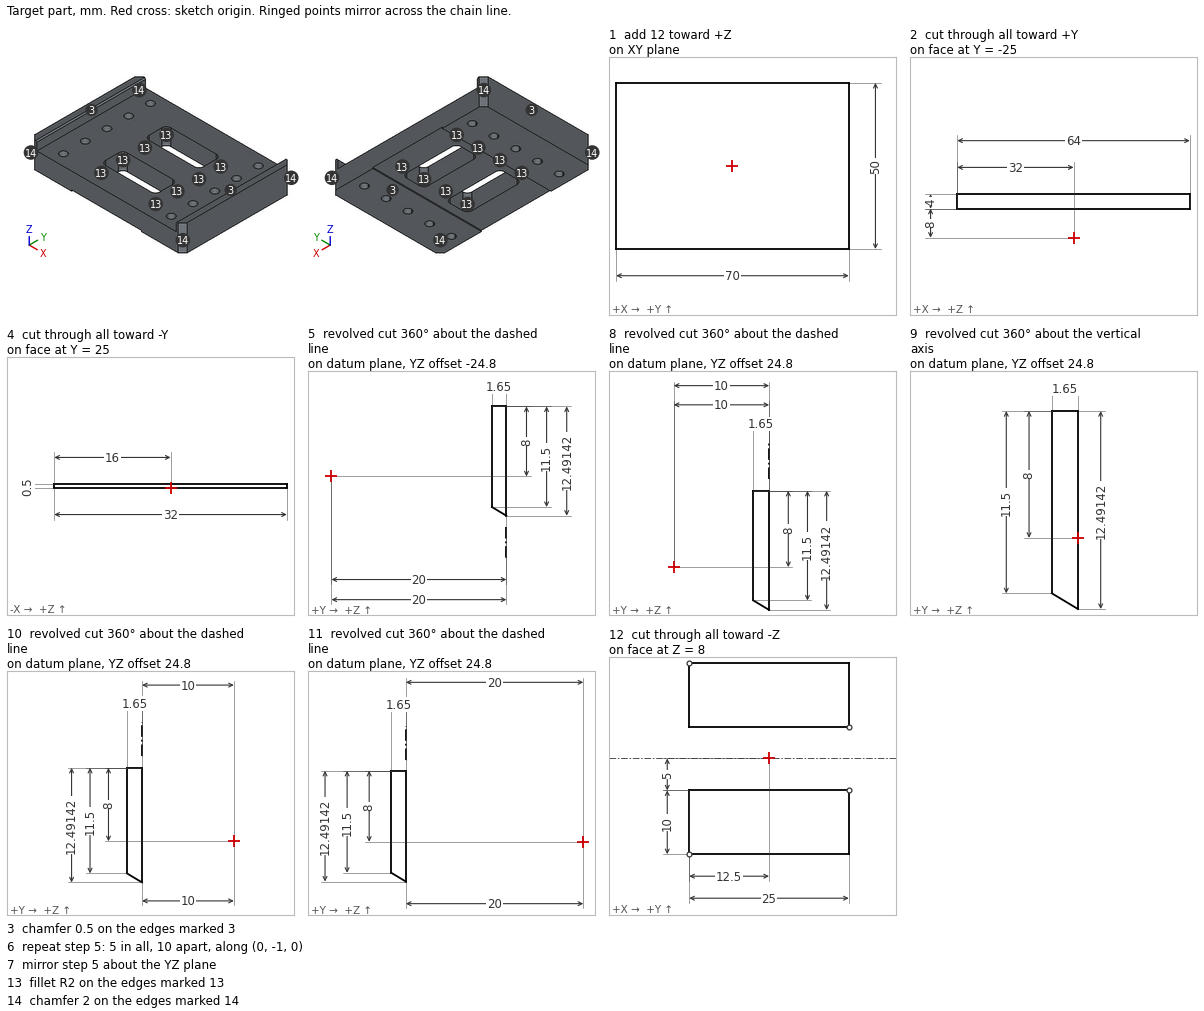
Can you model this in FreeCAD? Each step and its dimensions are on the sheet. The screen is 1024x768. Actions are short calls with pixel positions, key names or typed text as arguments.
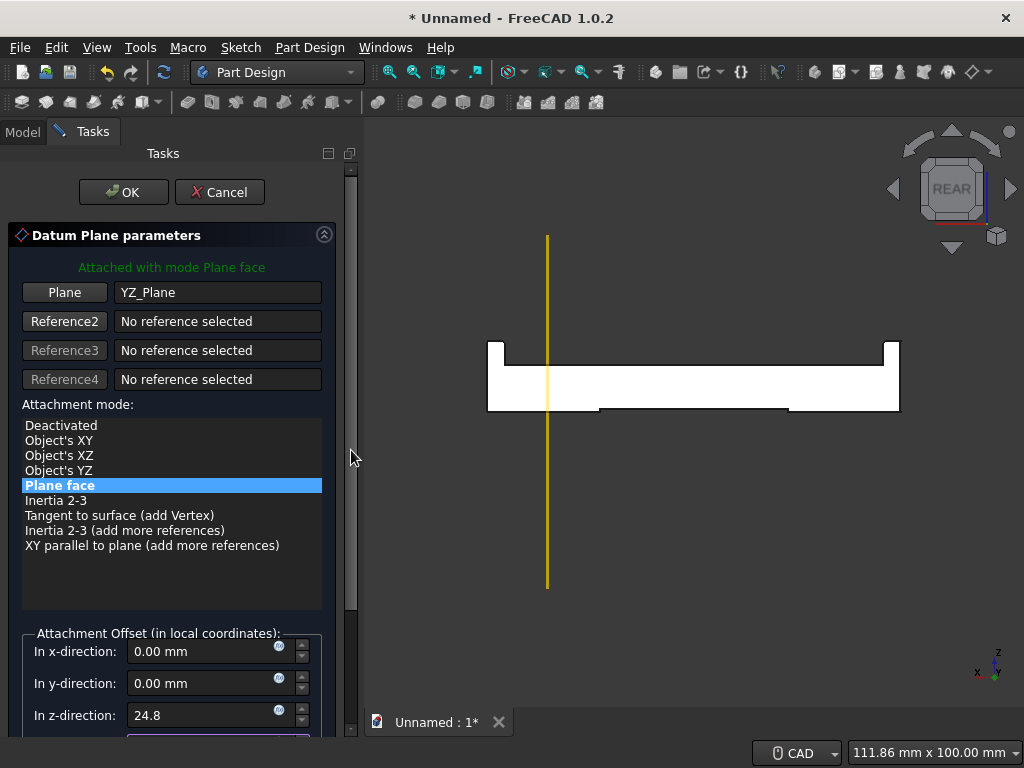
click(124, 192)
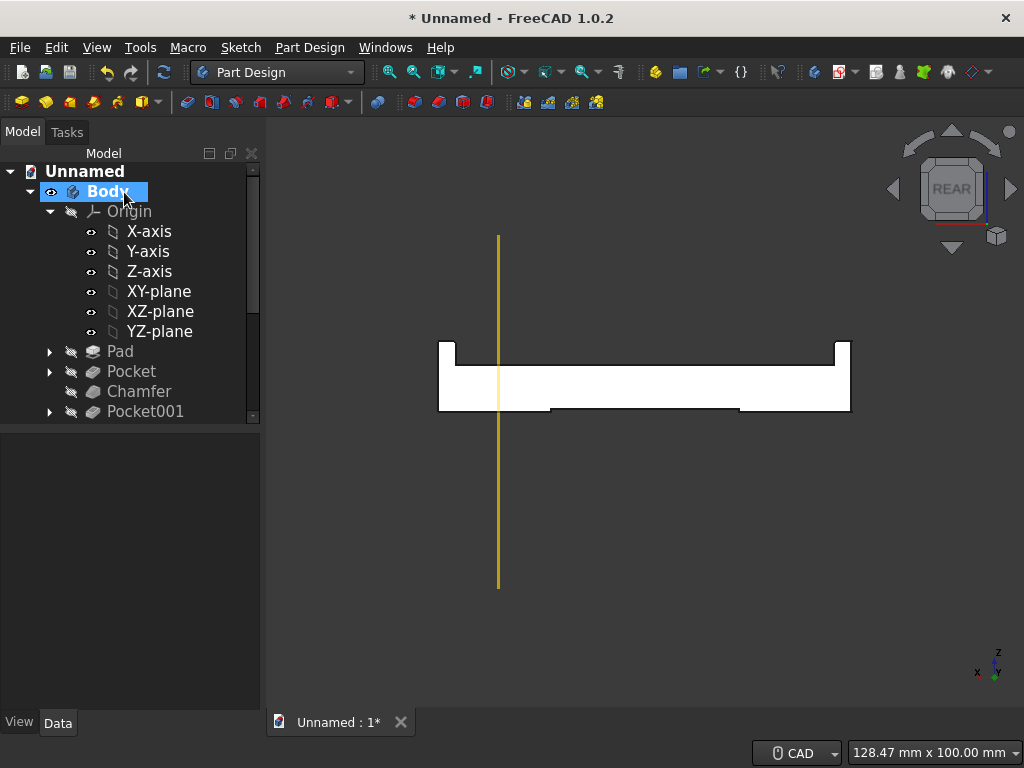
scroll(100, 287, down, 3)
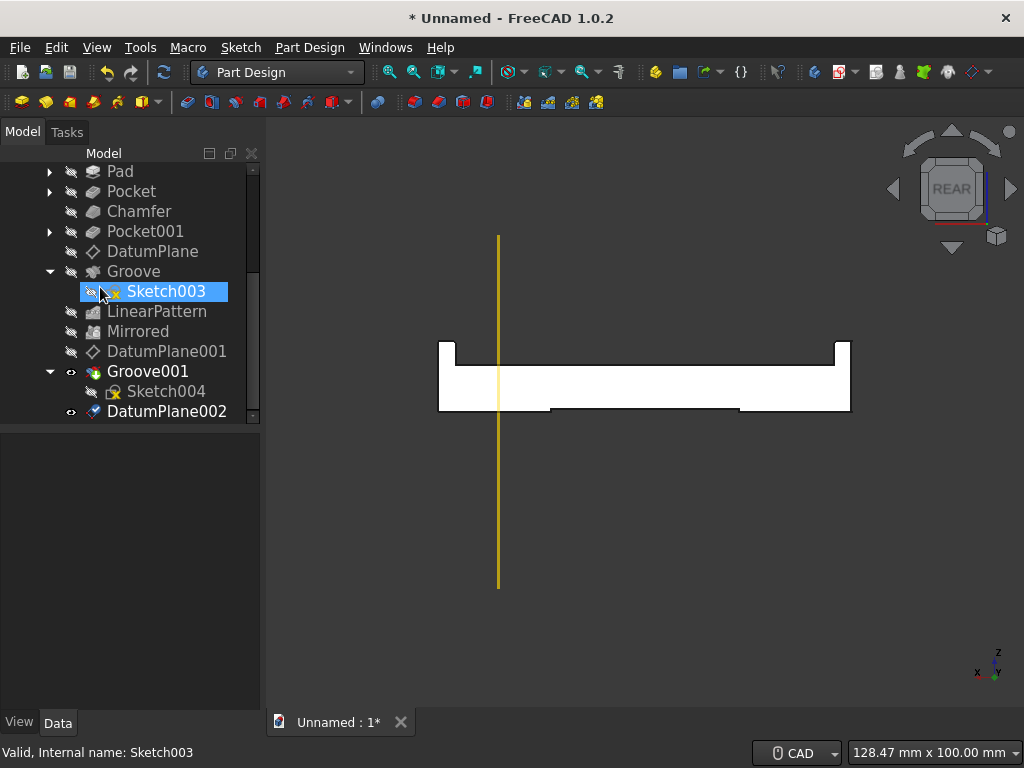
click(116, 412)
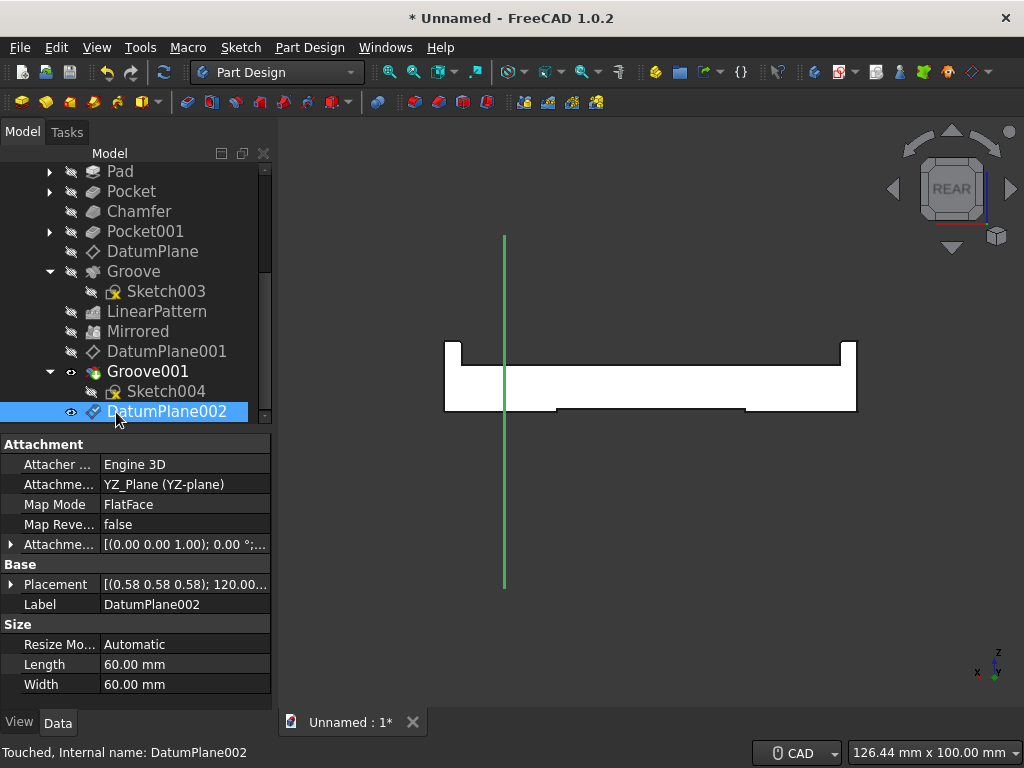
click(840, 72)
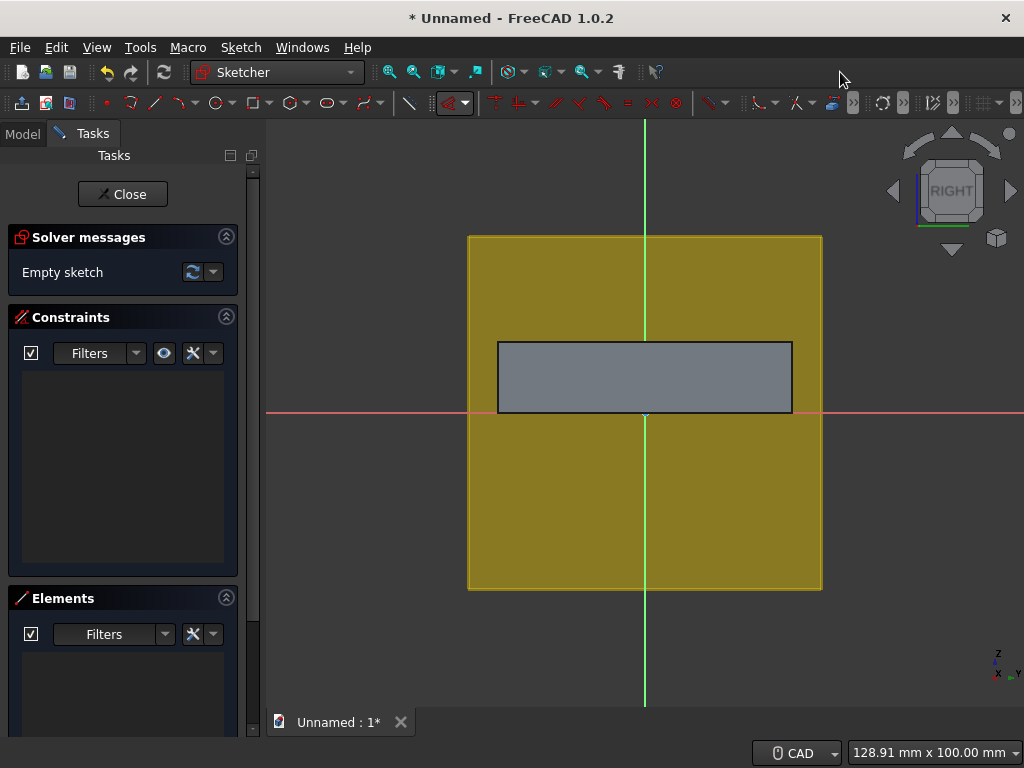
click(70, 104)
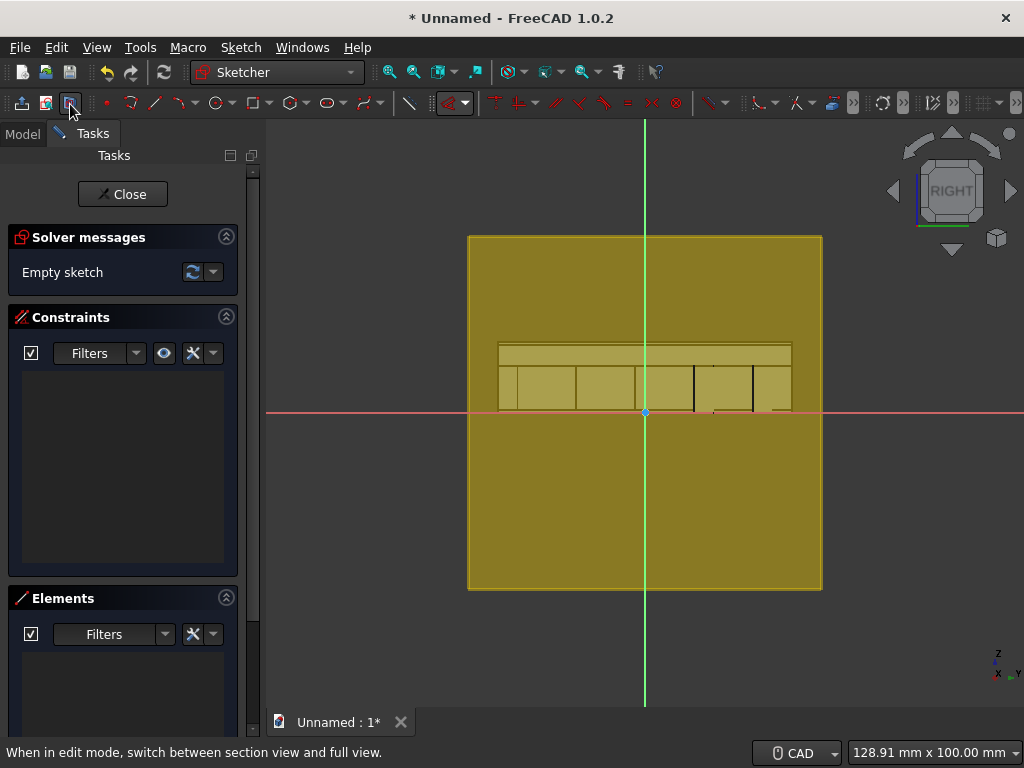
scroll(656, 400, up, 8)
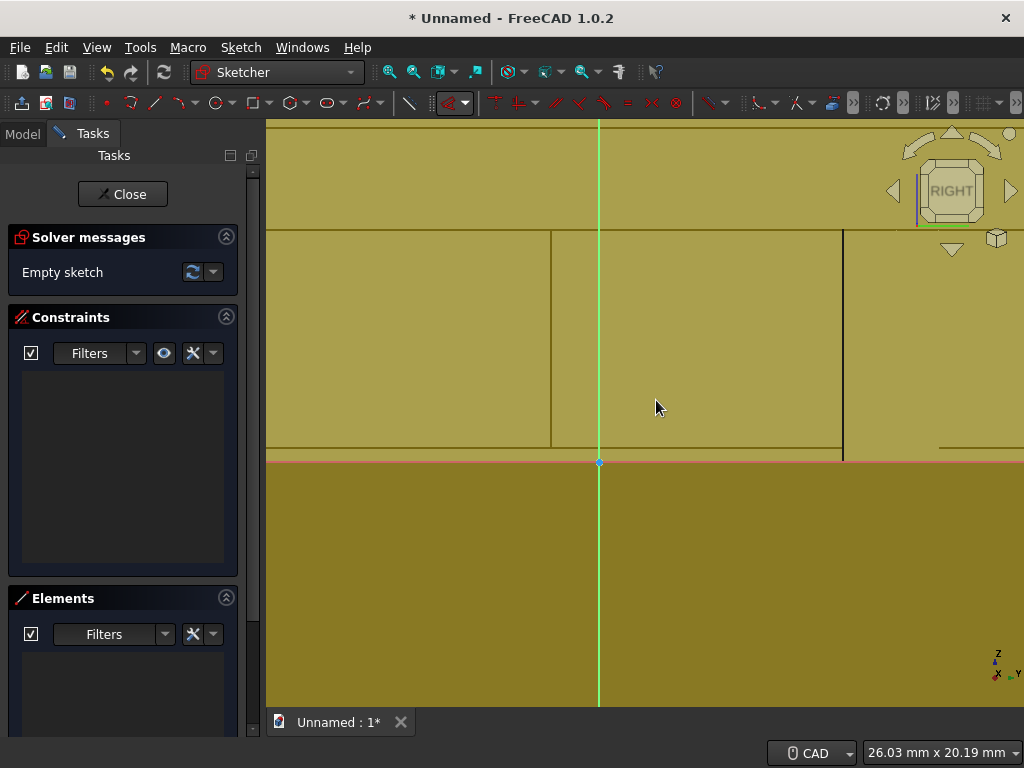
click(132, 104)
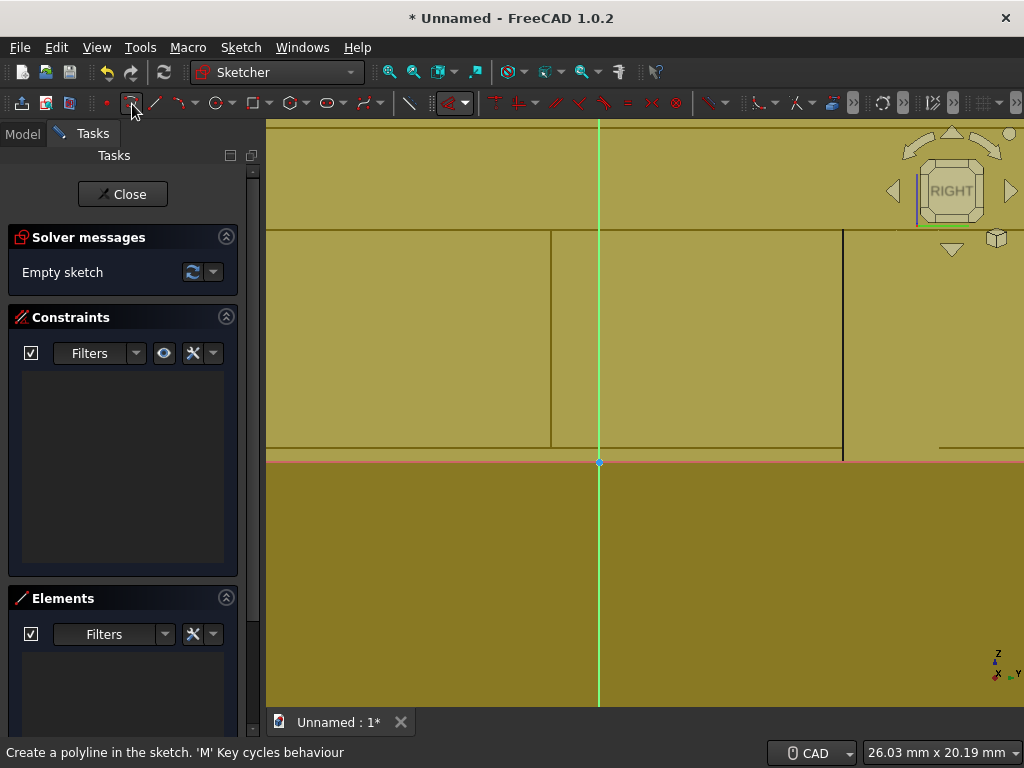
click(551, 564)
click(551, 230)
click(599, 230)
click(590, 593)
click(551, 565)
key(Escape)
key(Escape)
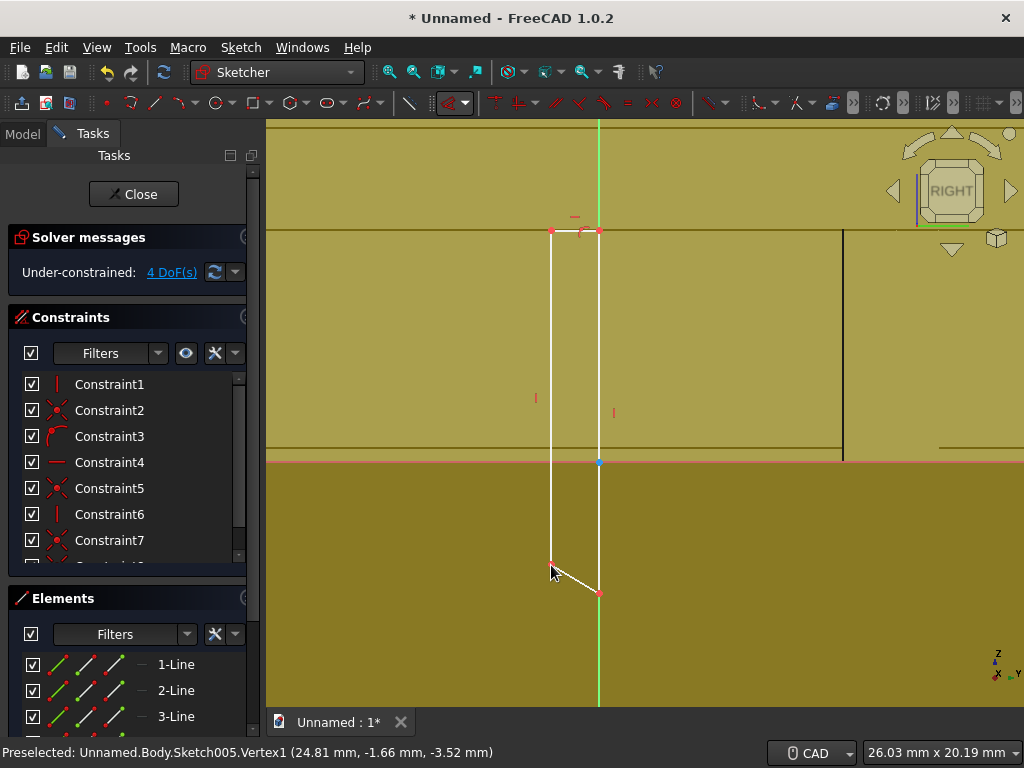
click(551, 231)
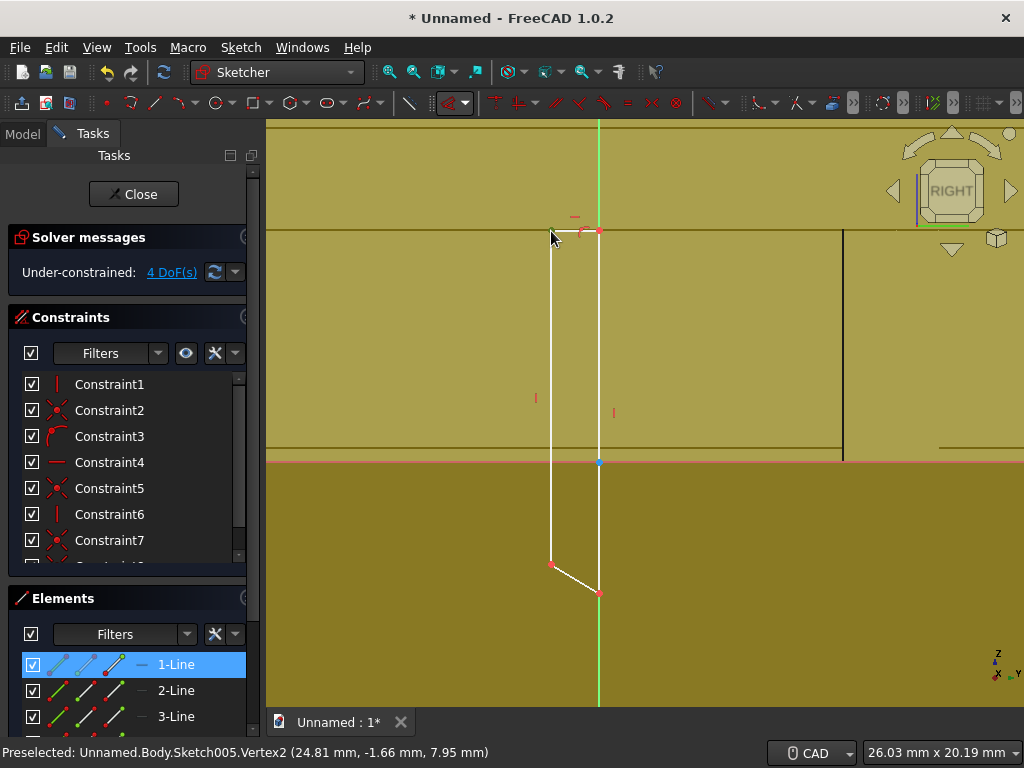
key(i)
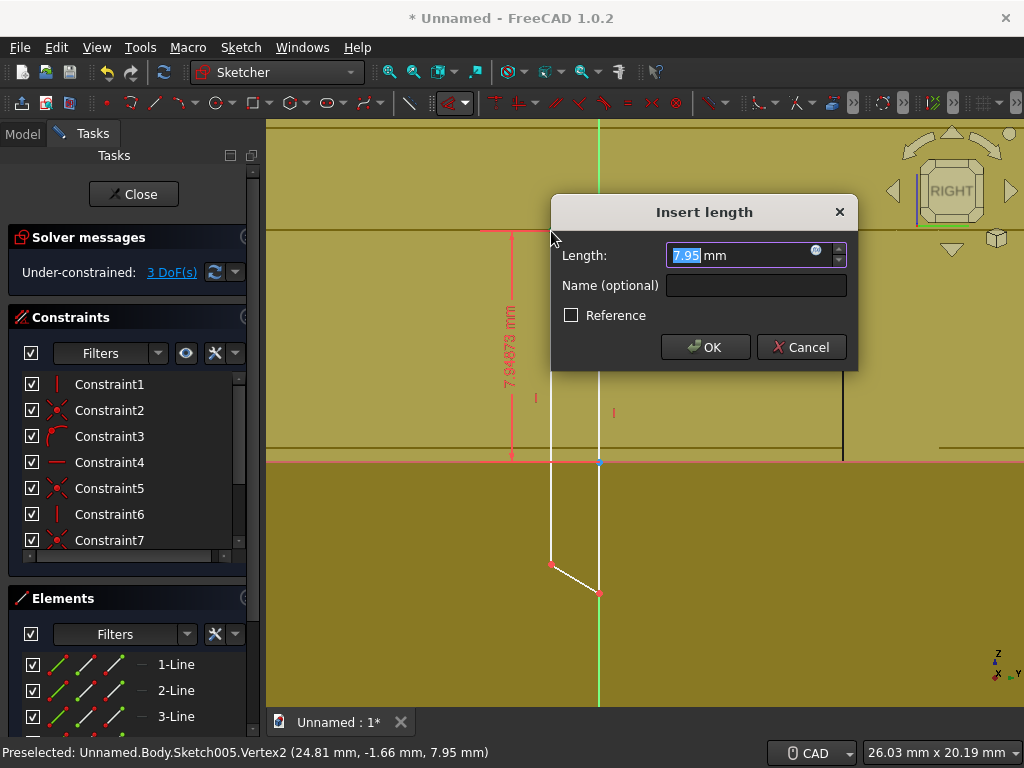
text(8)
key(Return)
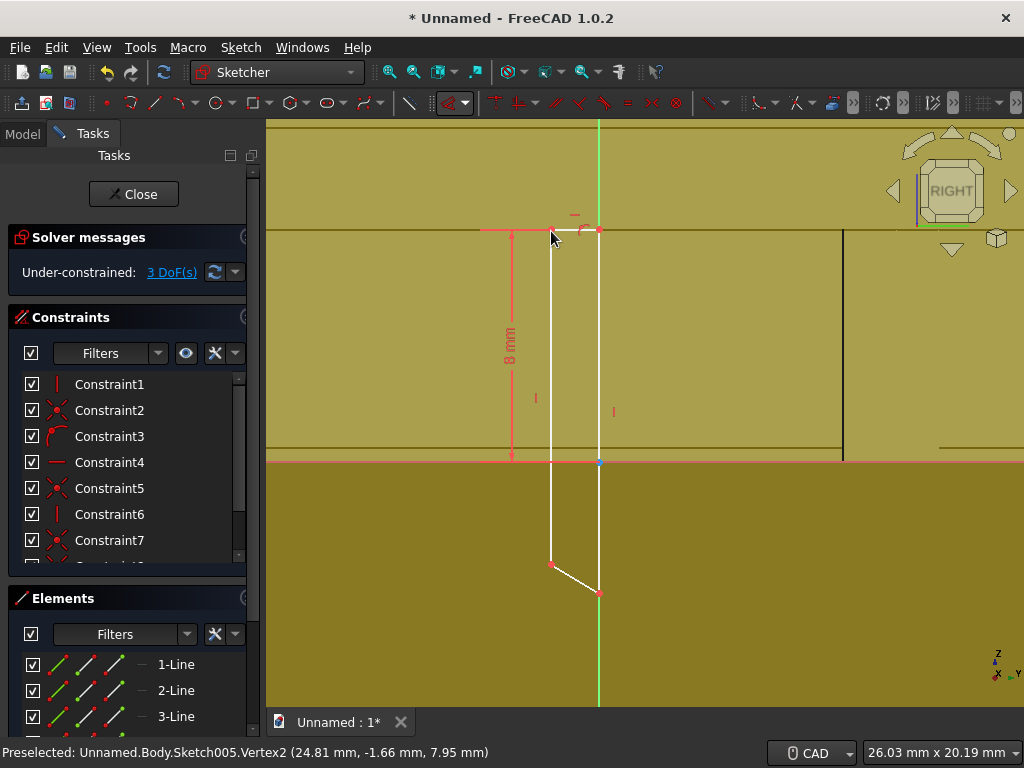
click(551, 464)